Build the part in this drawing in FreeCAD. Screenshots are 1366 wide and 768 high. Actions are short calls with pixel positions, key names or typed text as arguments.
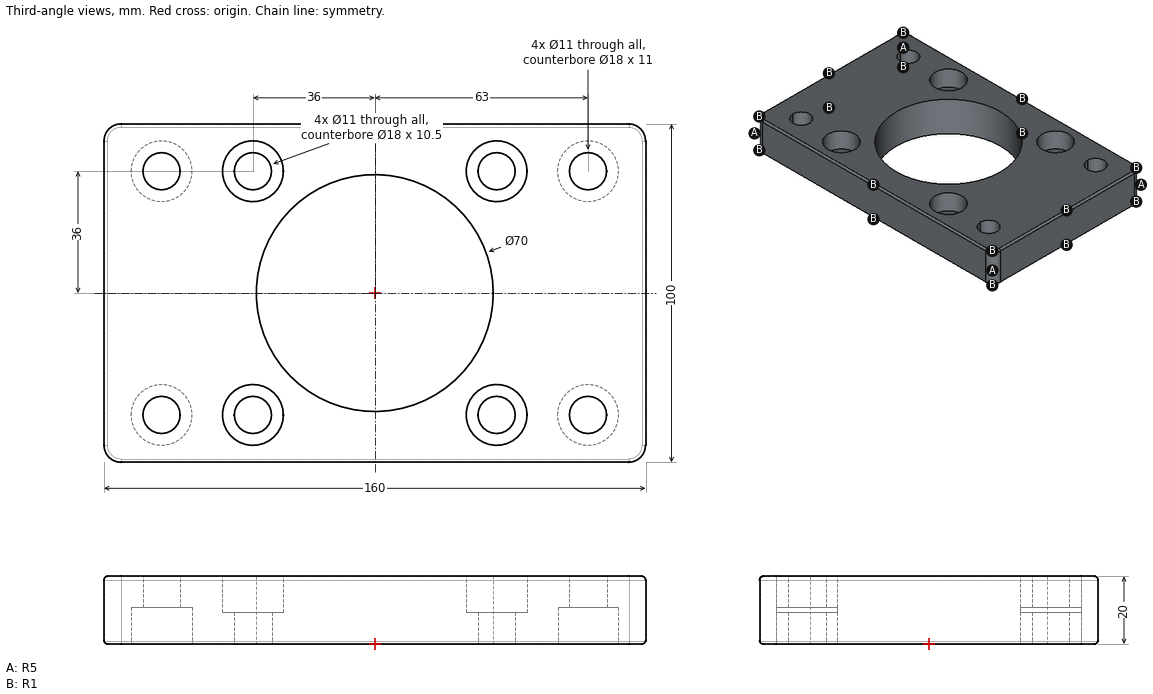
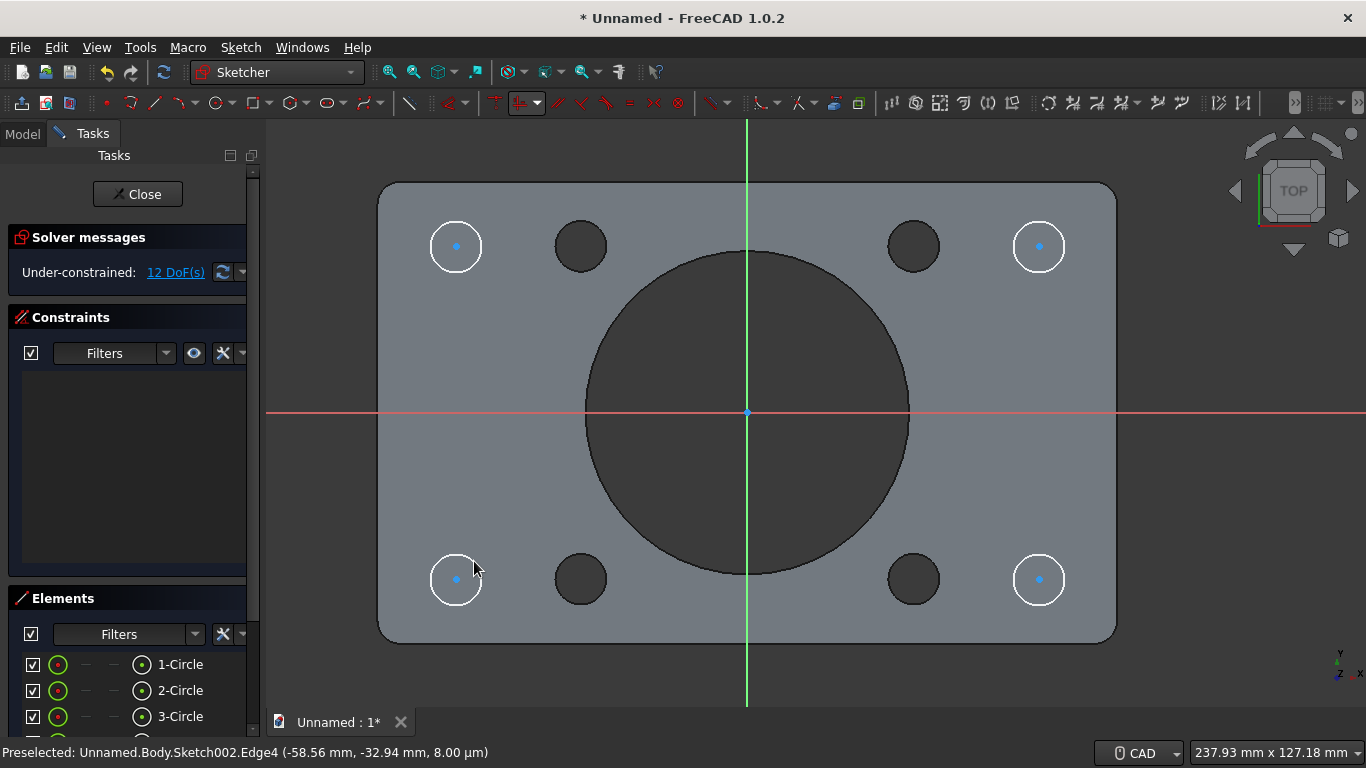
click(1057, 229)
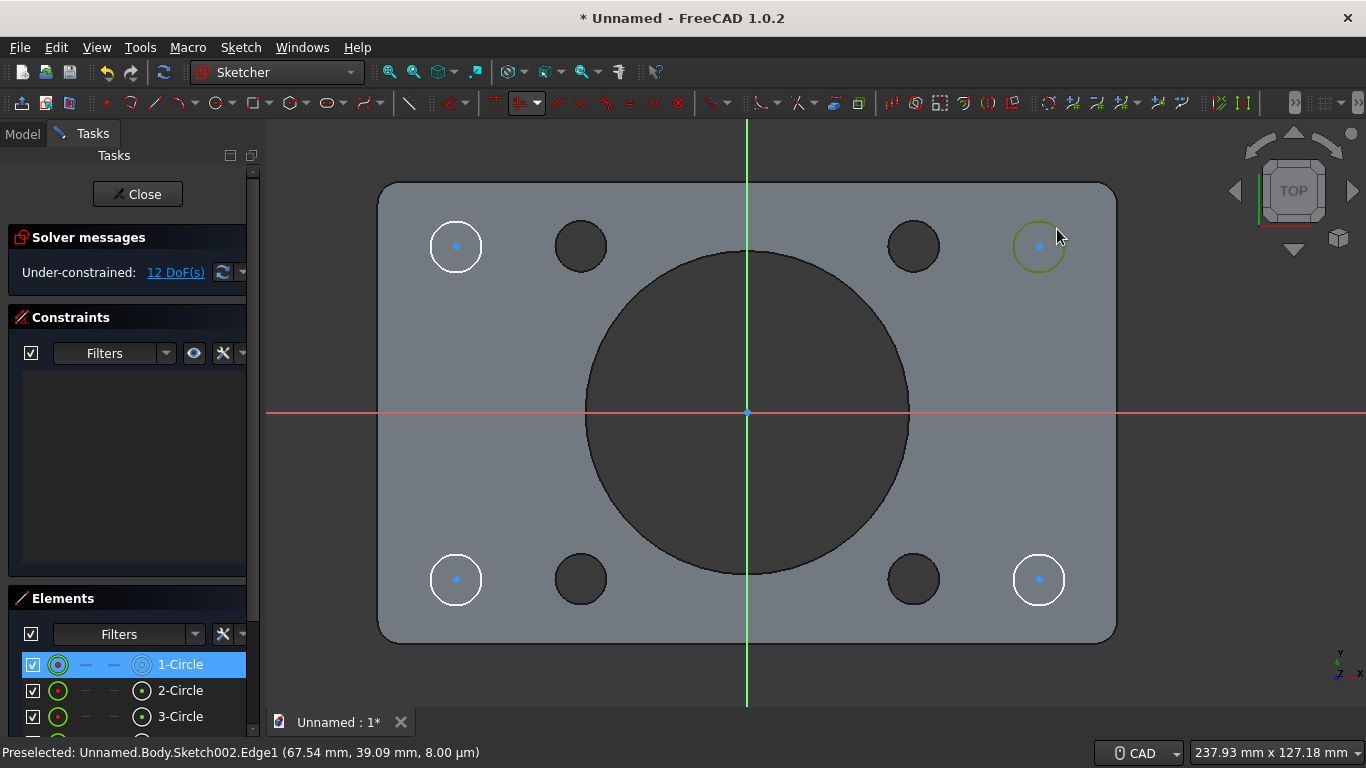
click(474, 229)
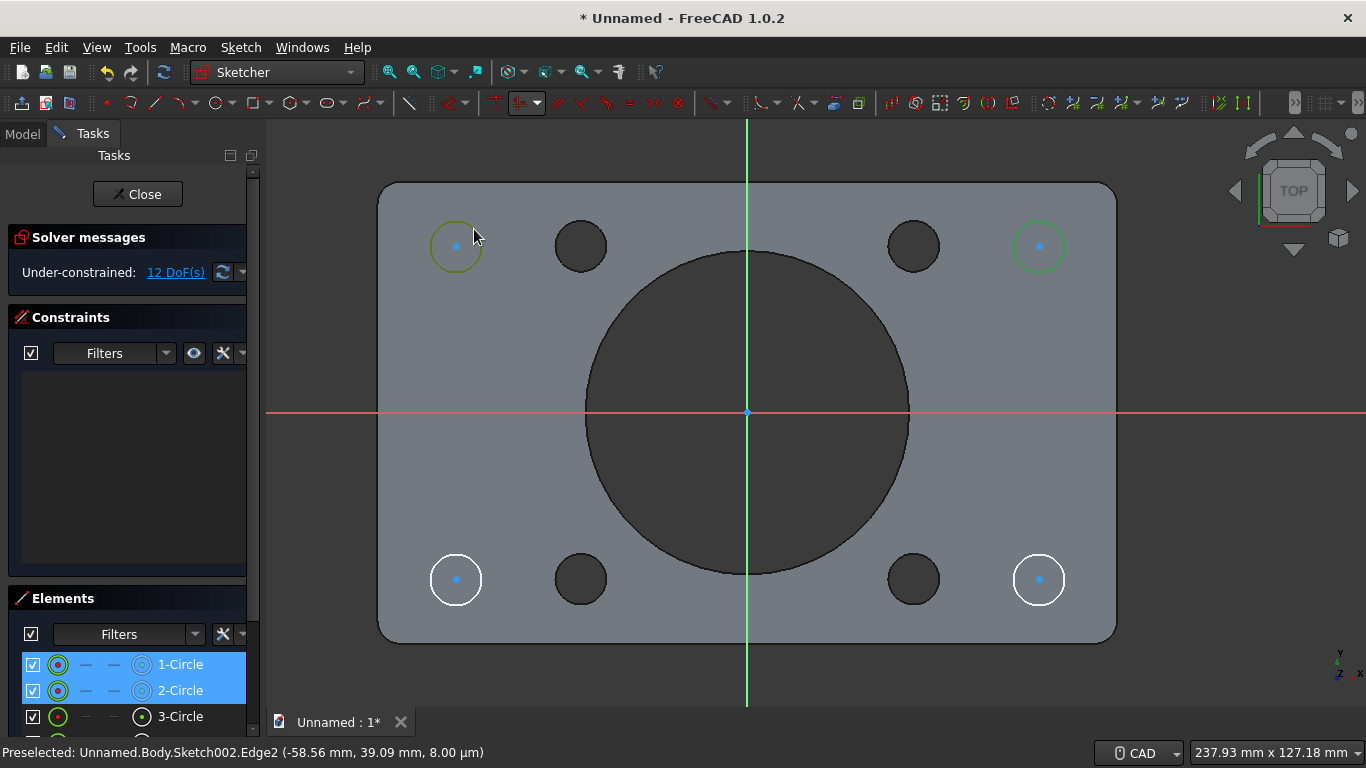
click(1057, 562)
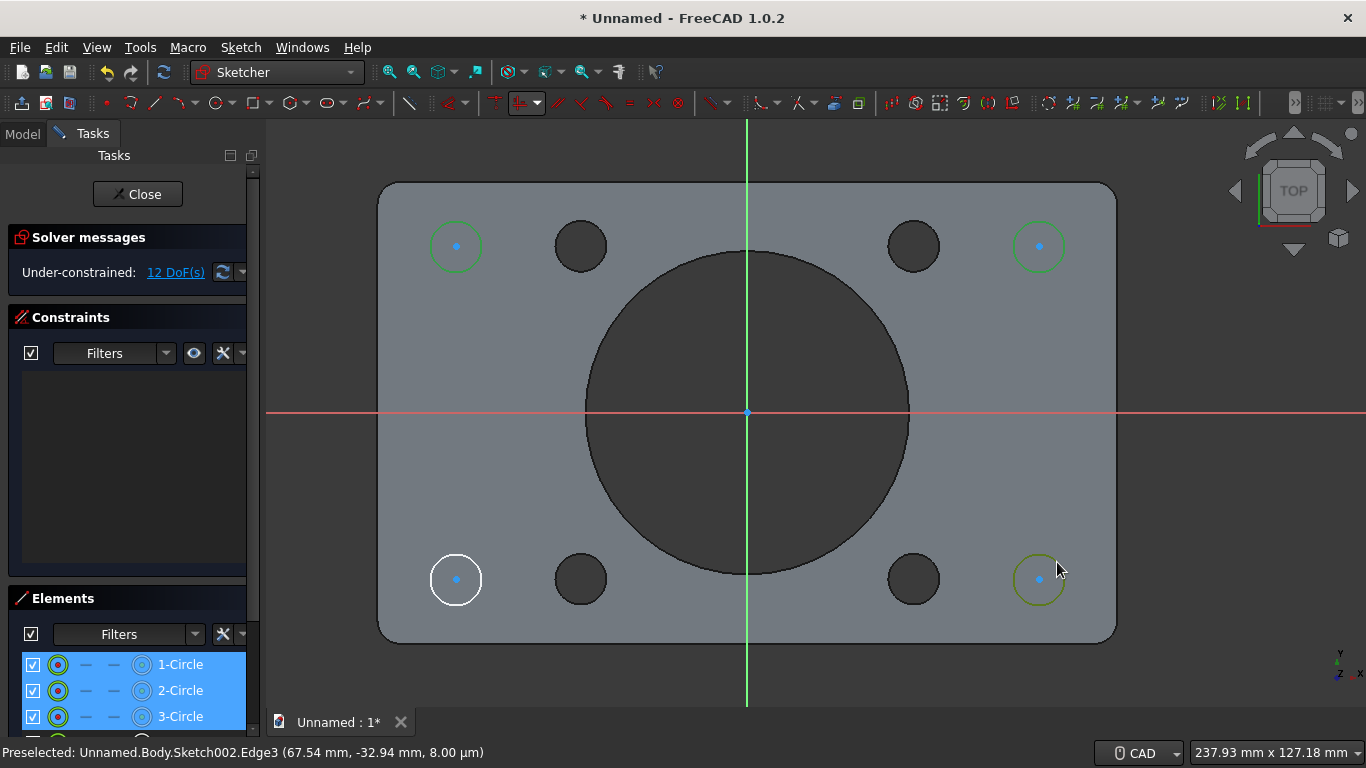
click(474, 562)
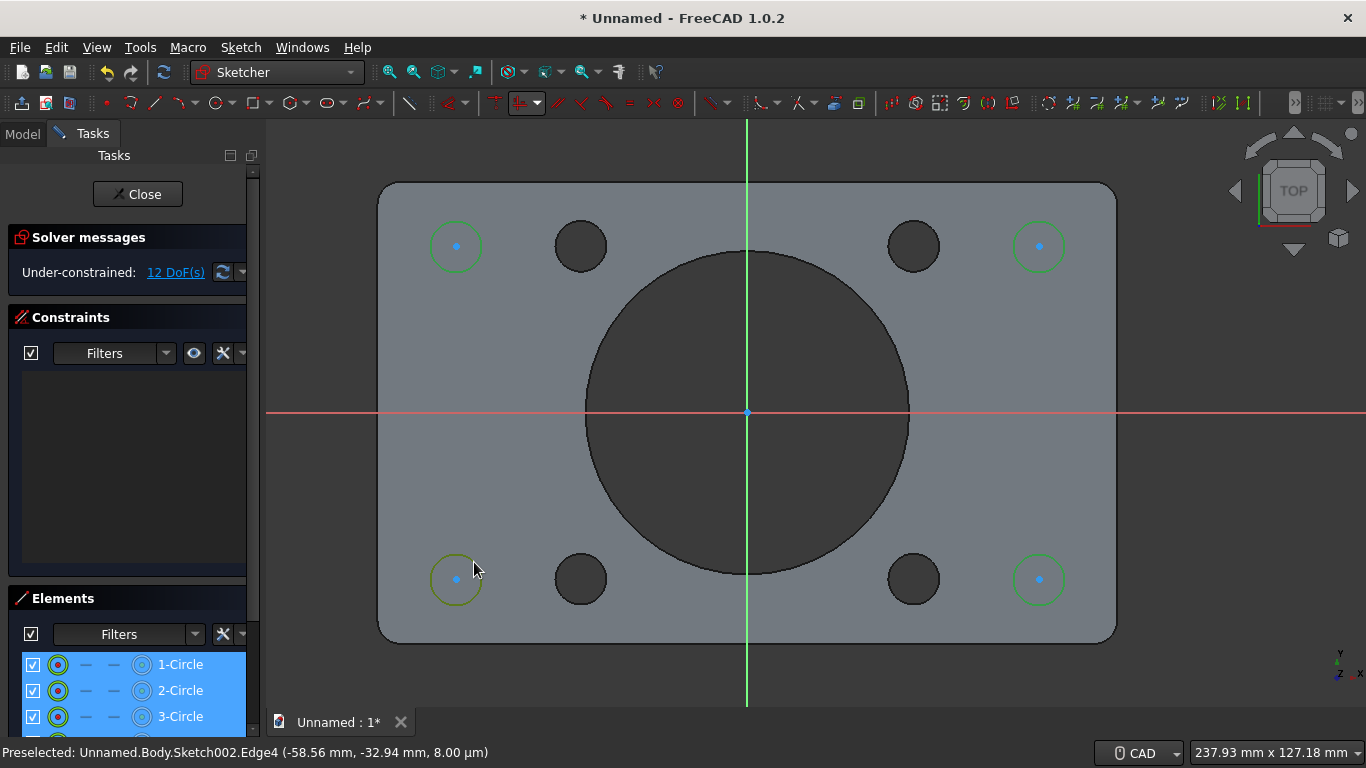
key(e)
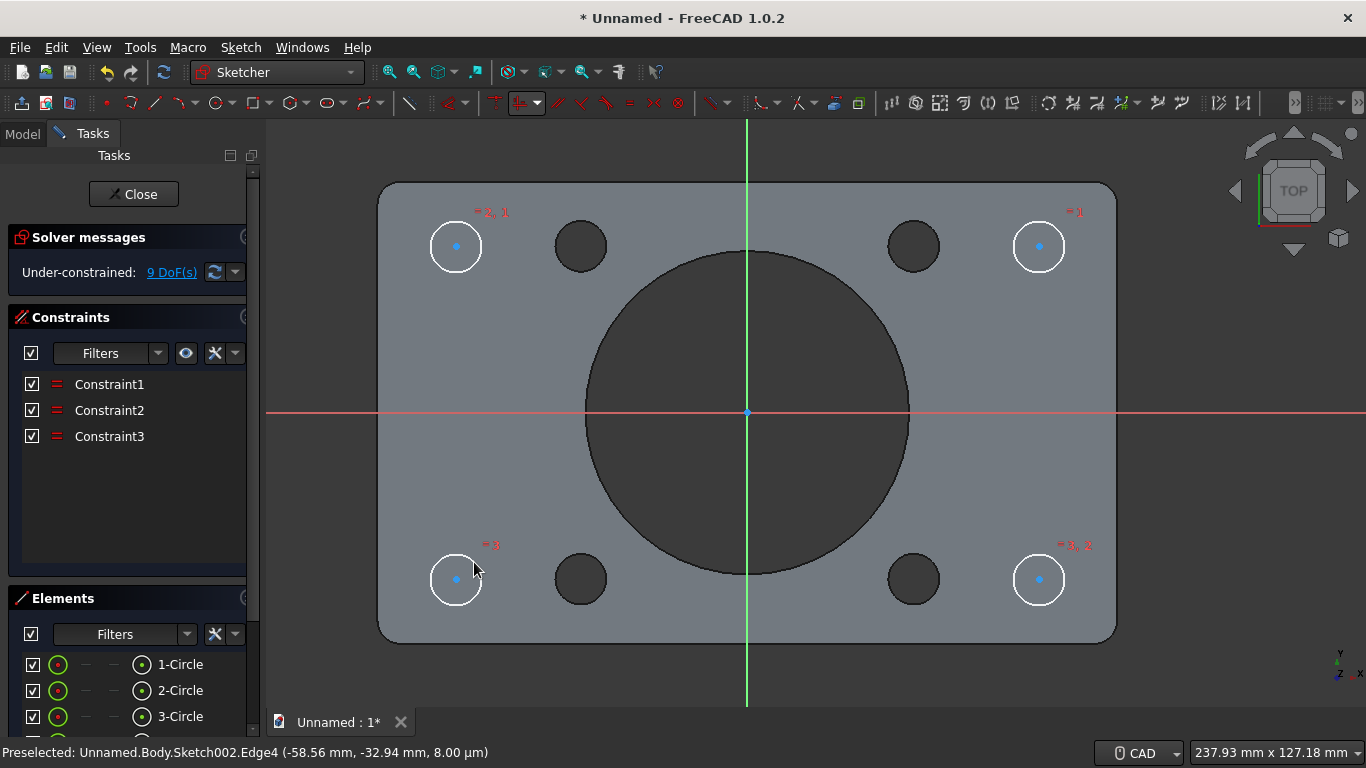
click(1039, 247)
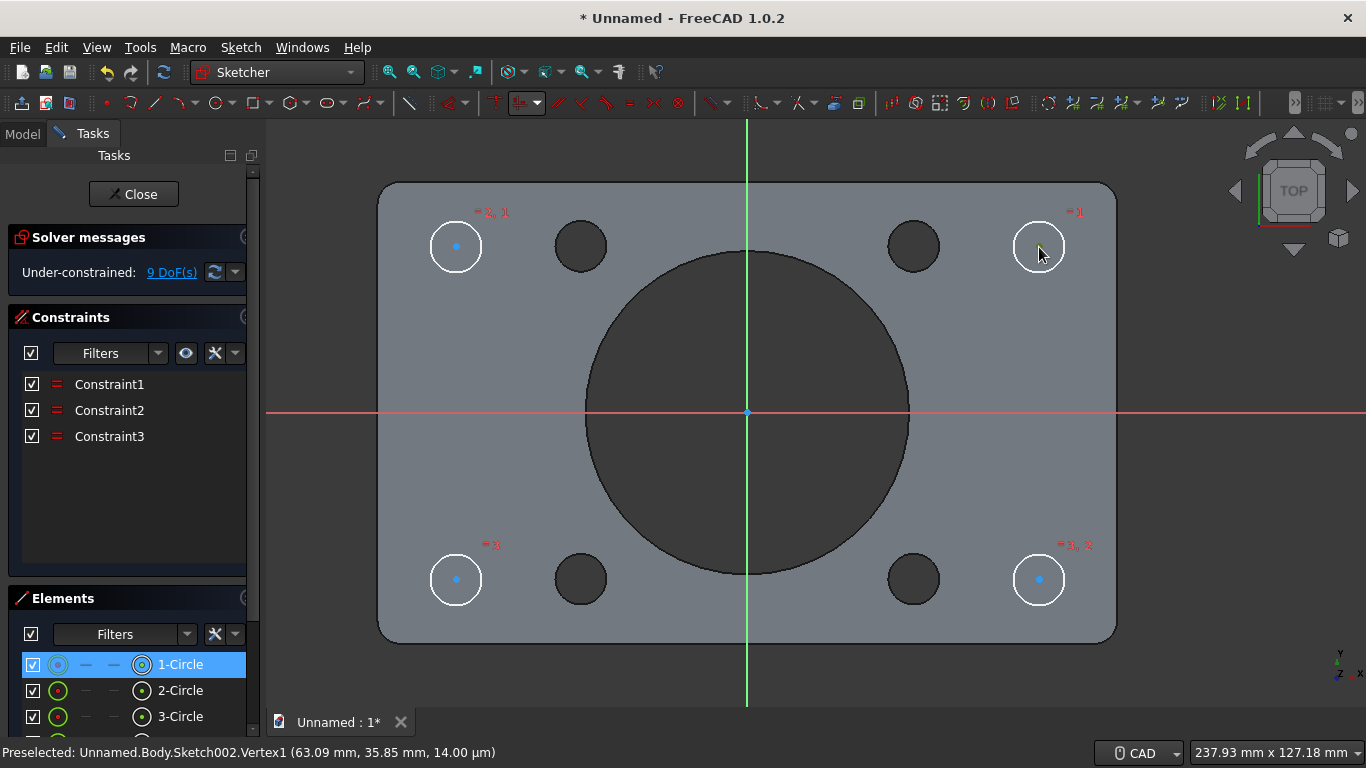
click(456, 247)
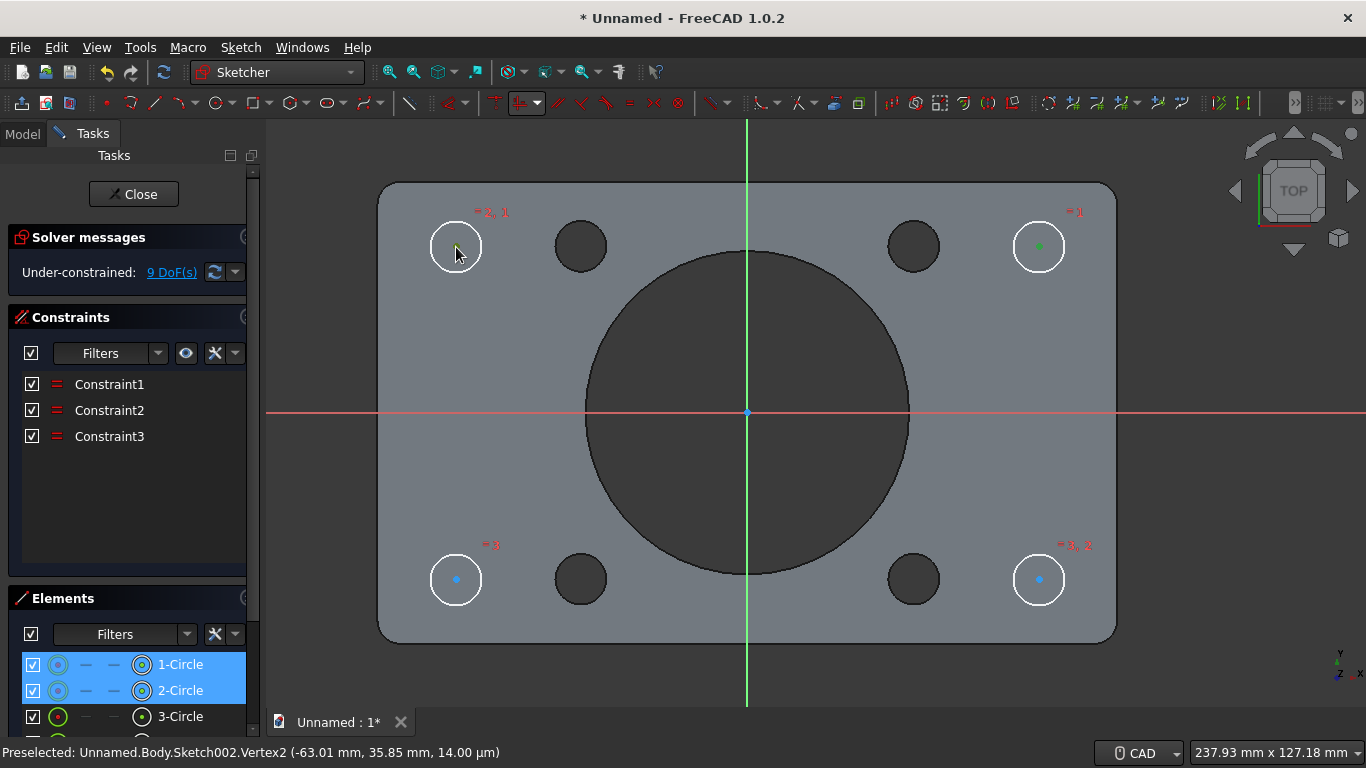
click(747, 641)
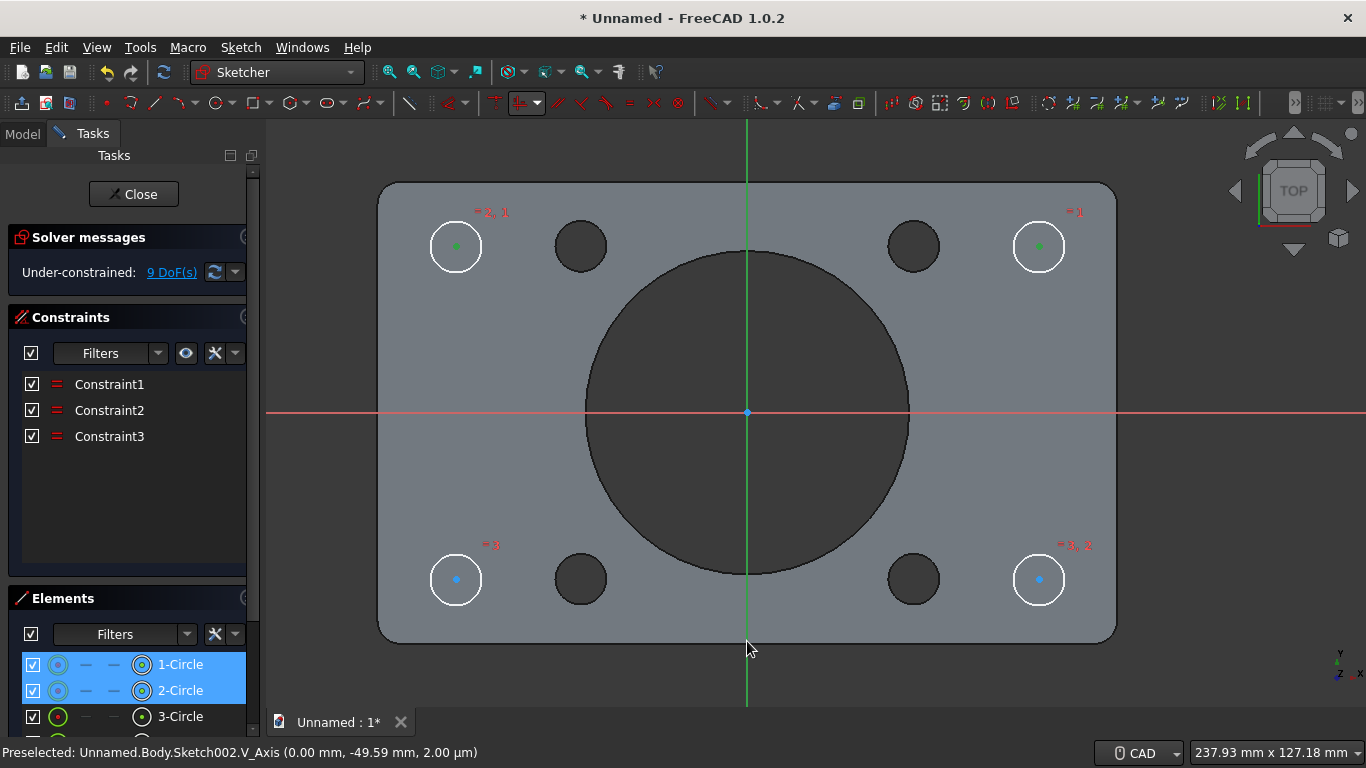
key(s)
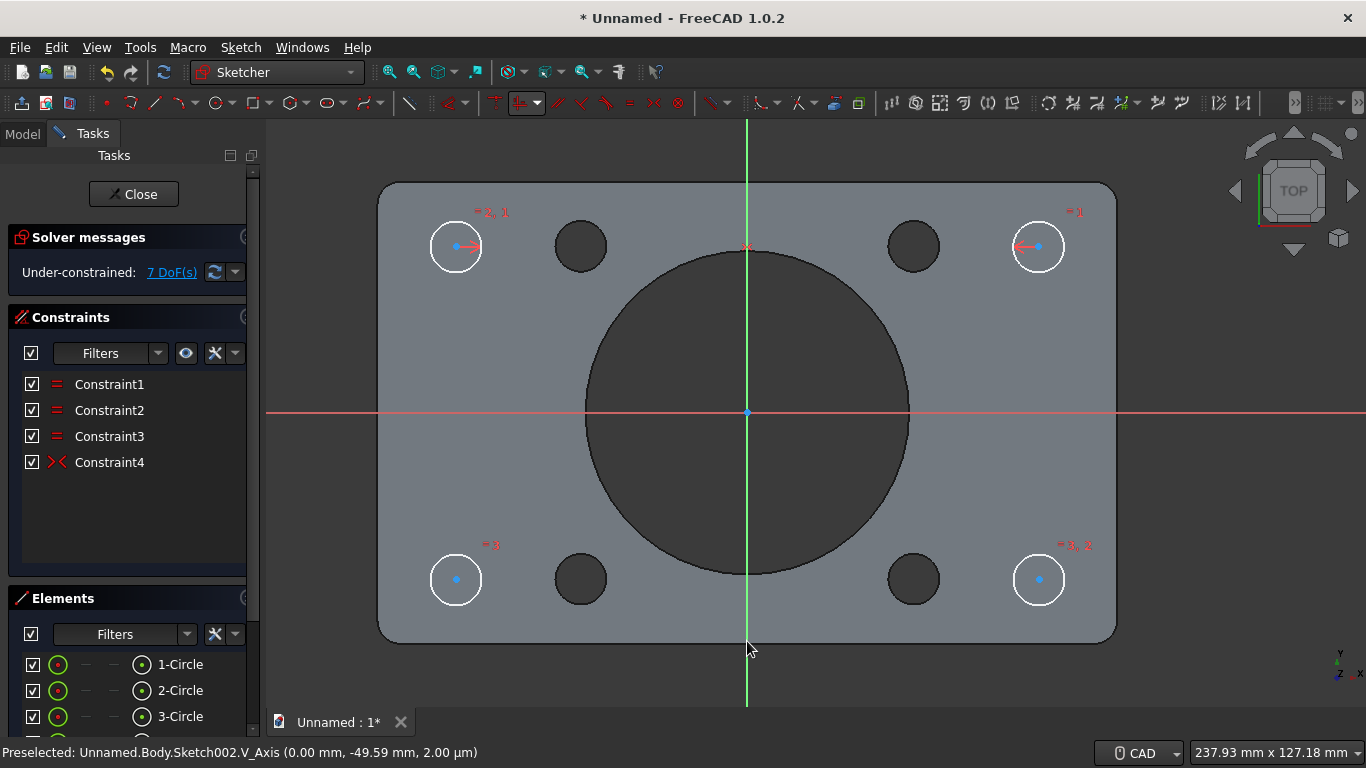
click(1039, 247)